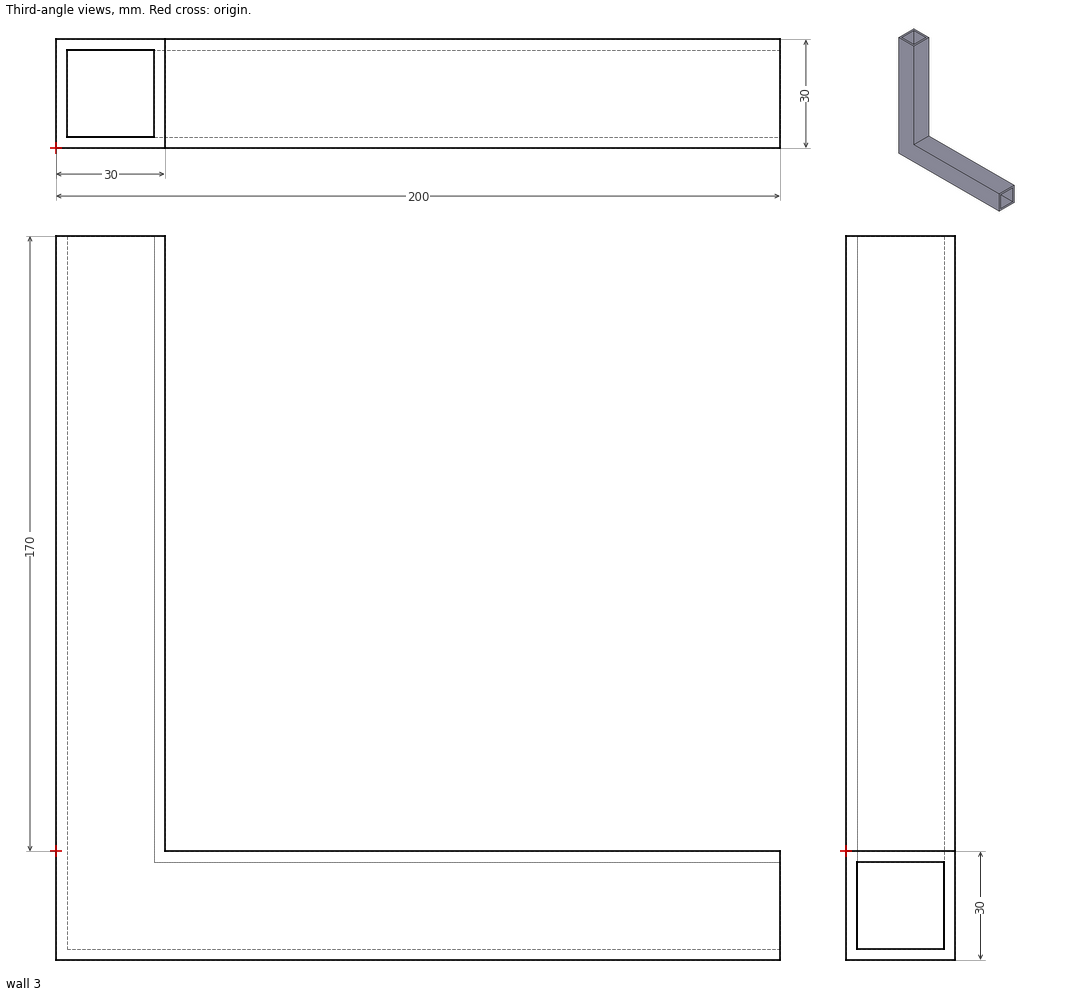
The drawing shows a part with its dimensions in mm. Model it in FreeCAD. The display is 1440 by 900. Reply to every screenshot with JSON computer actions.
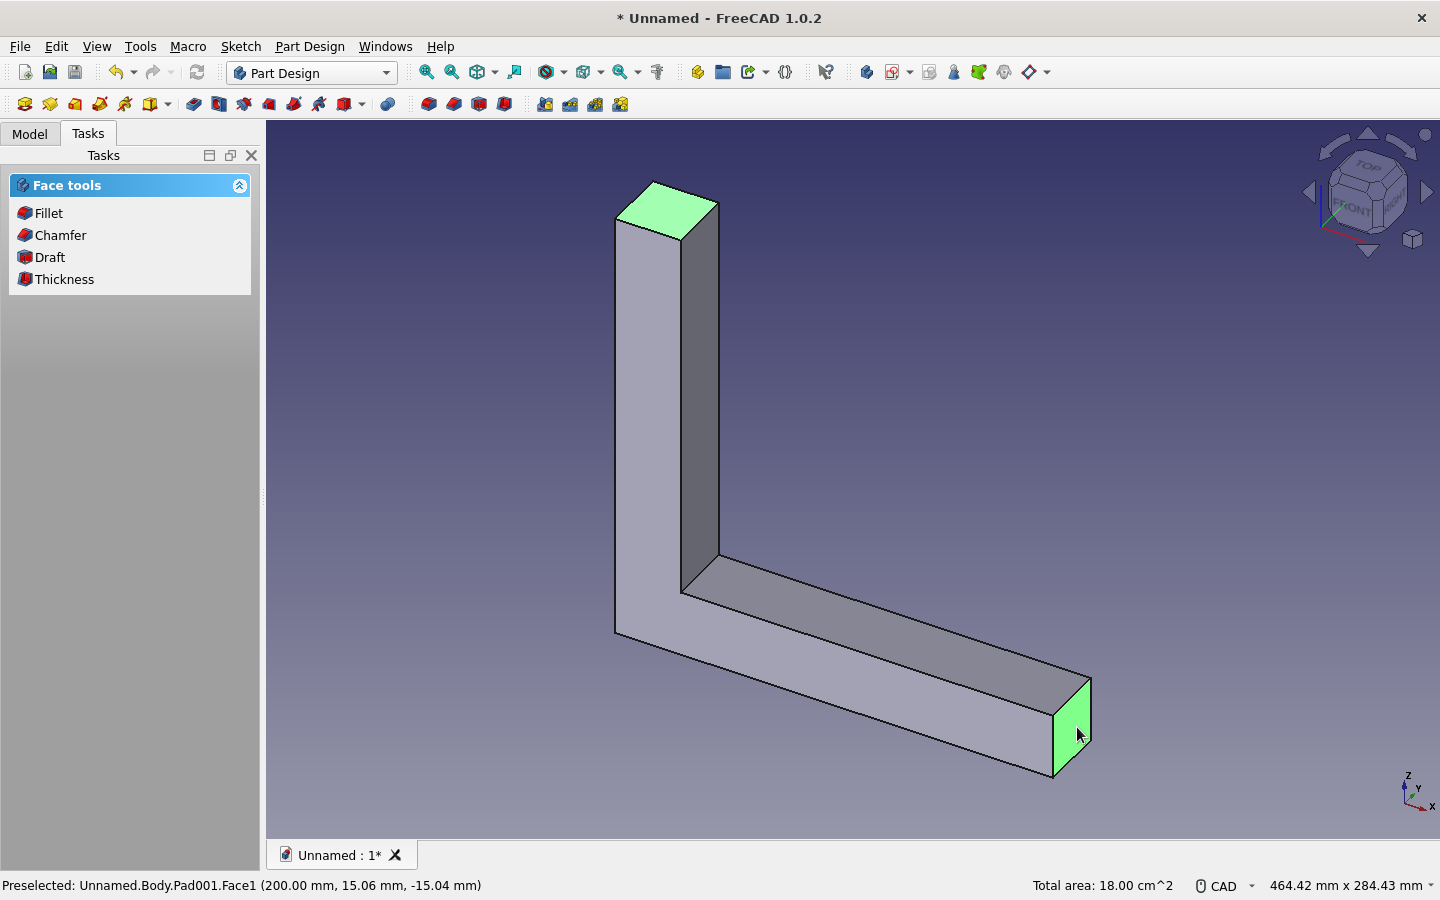
{"action": "left_click", "coordinate": [504, 104]}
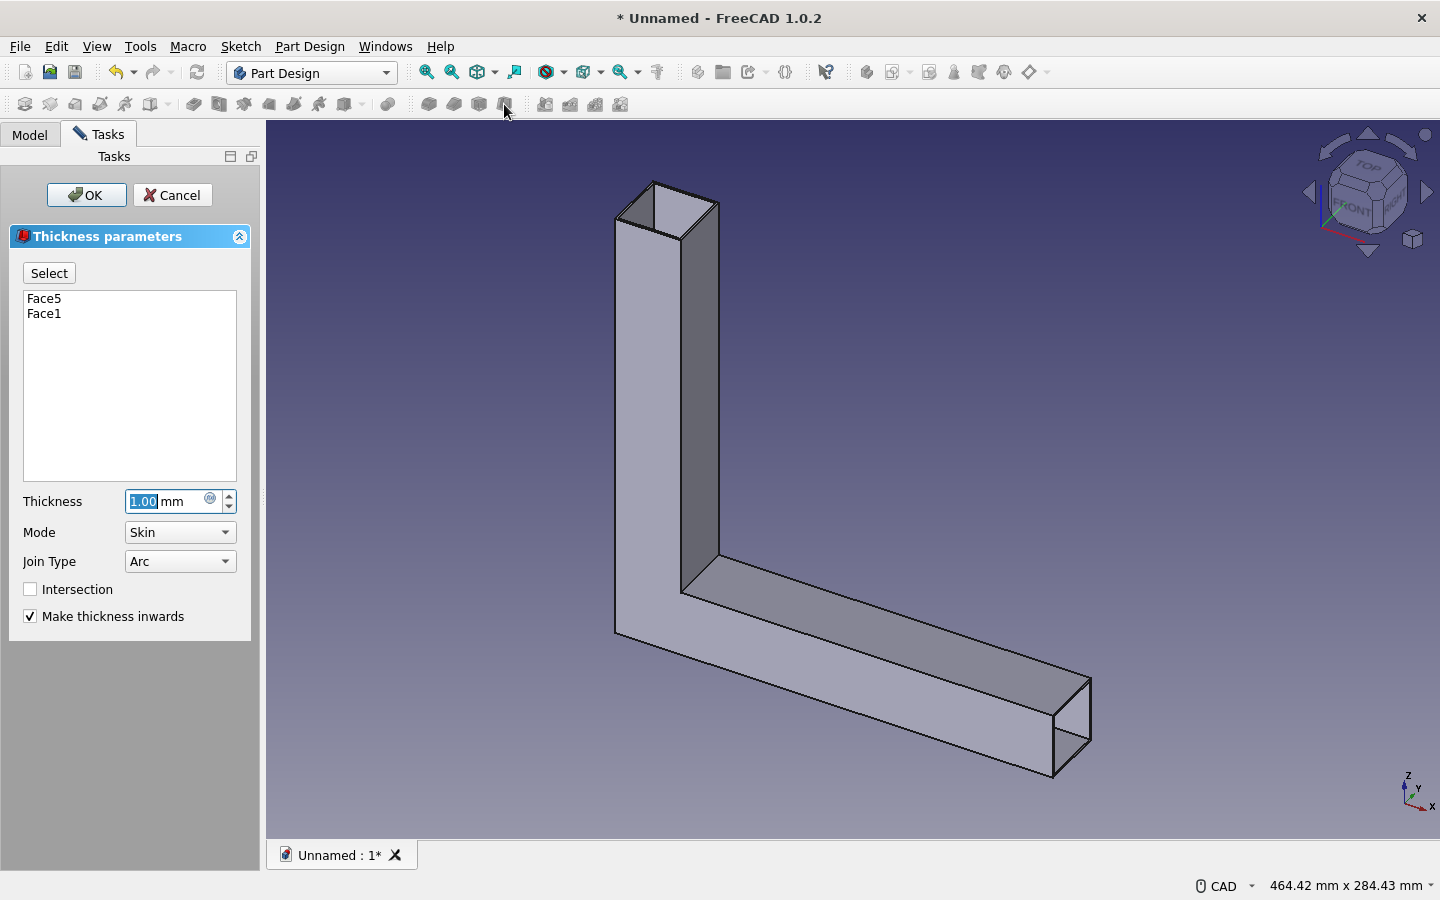
{"action": "type", "text": "3"}
{"action": "key", "text": "Tab"}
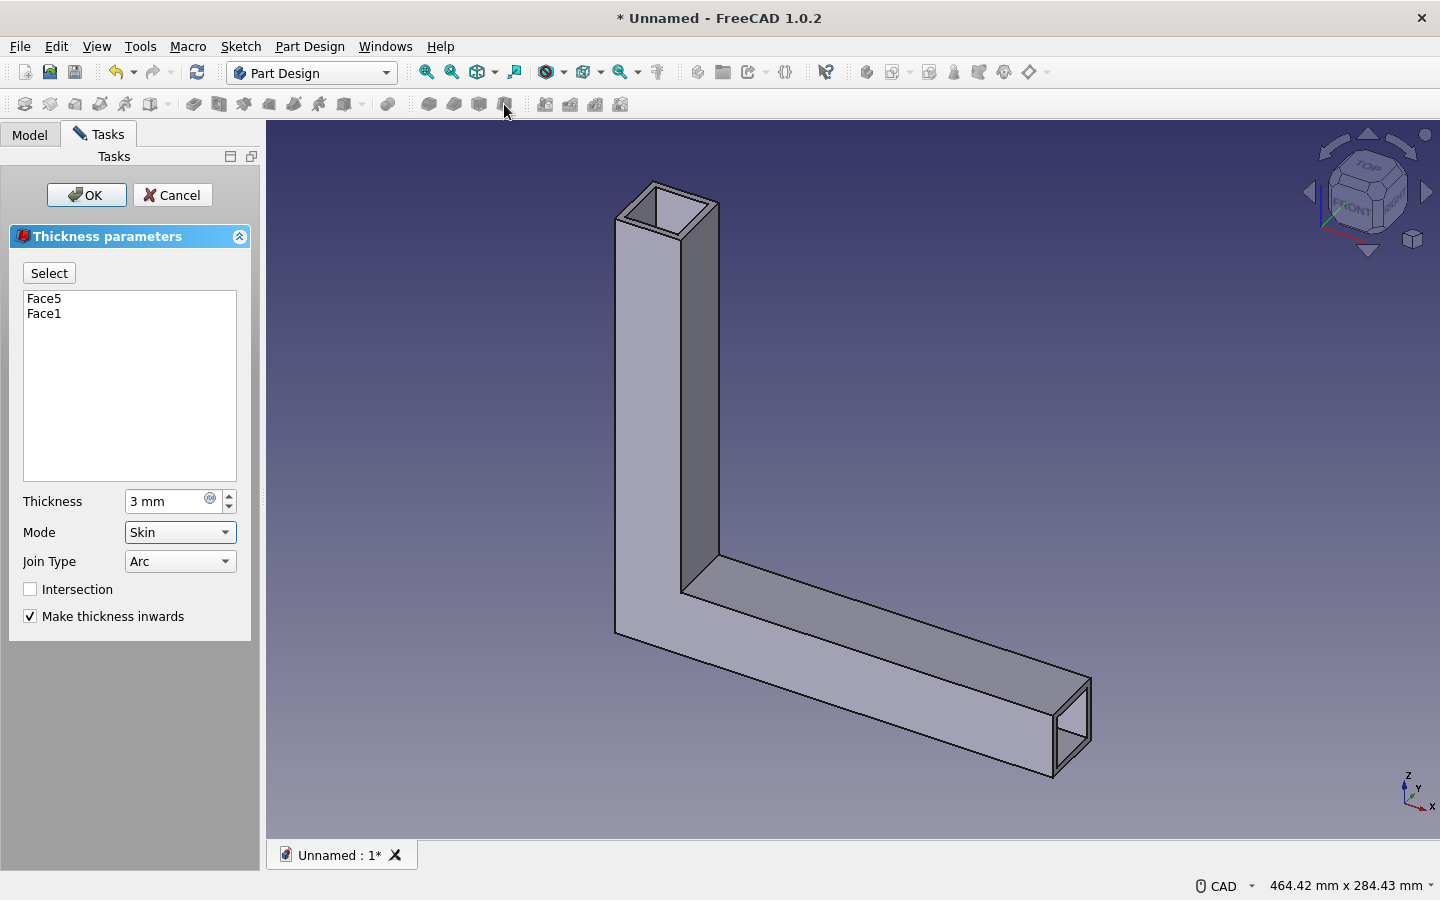
{"action": "left_click", "coordinate": [181, 562]}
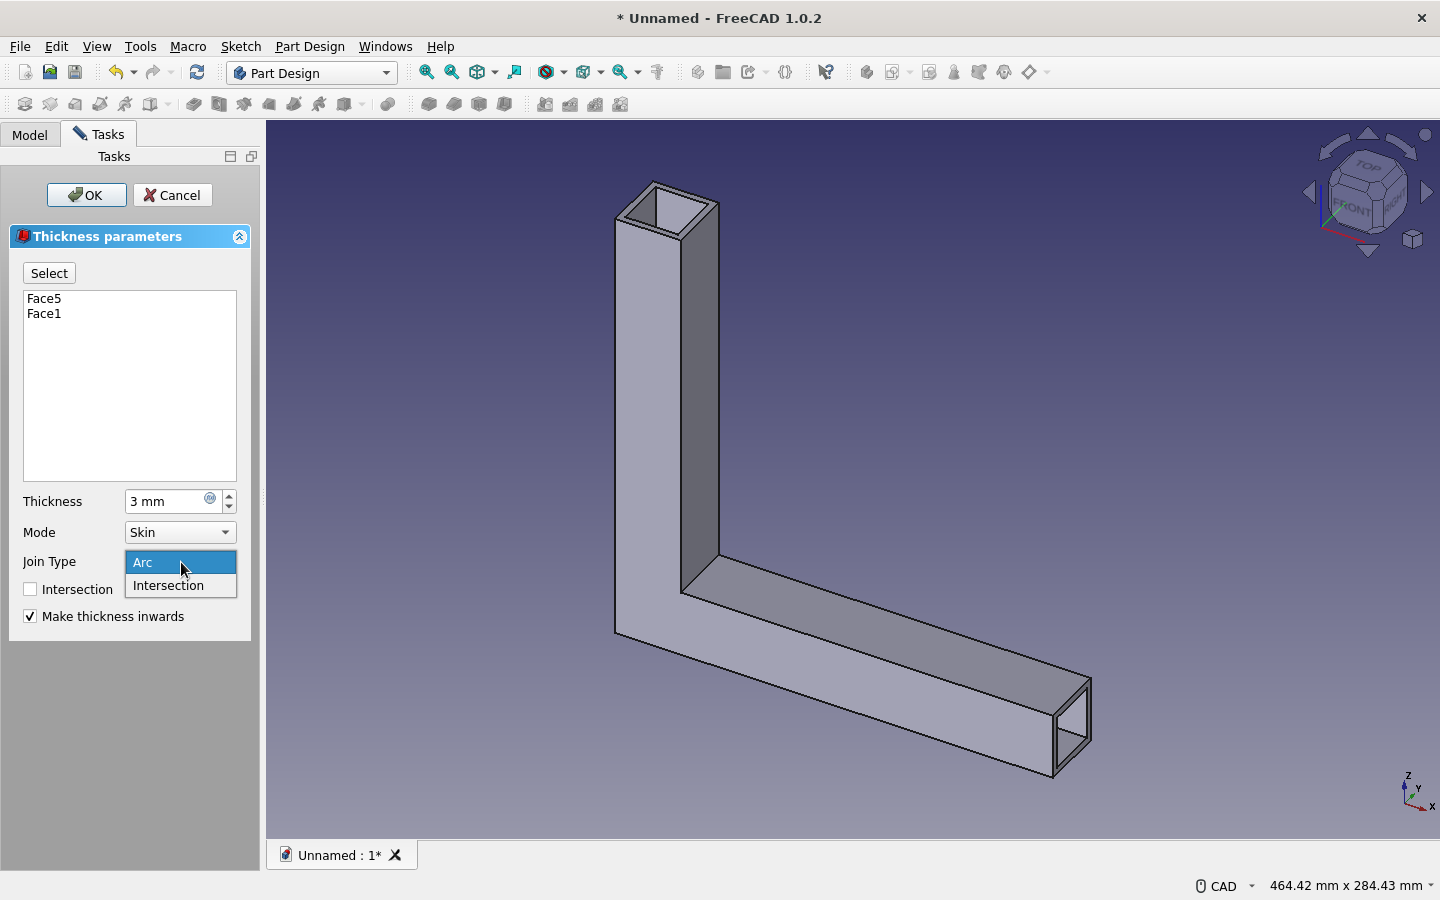
{"action": "left_click", "coordinate": [179, 586]}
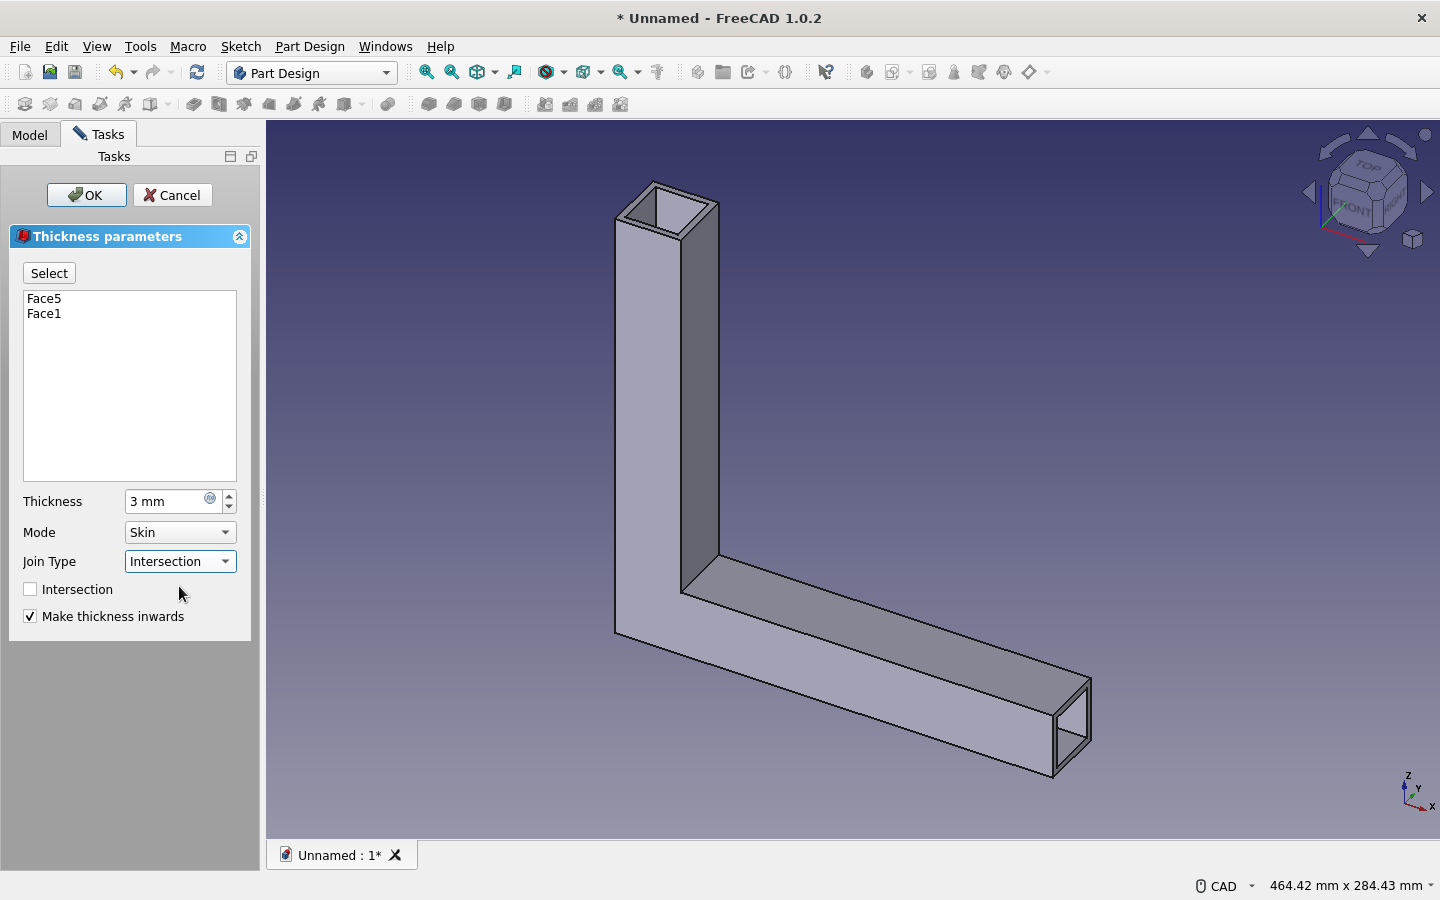
{"action": "left_click", "coordinate": [87, 195]}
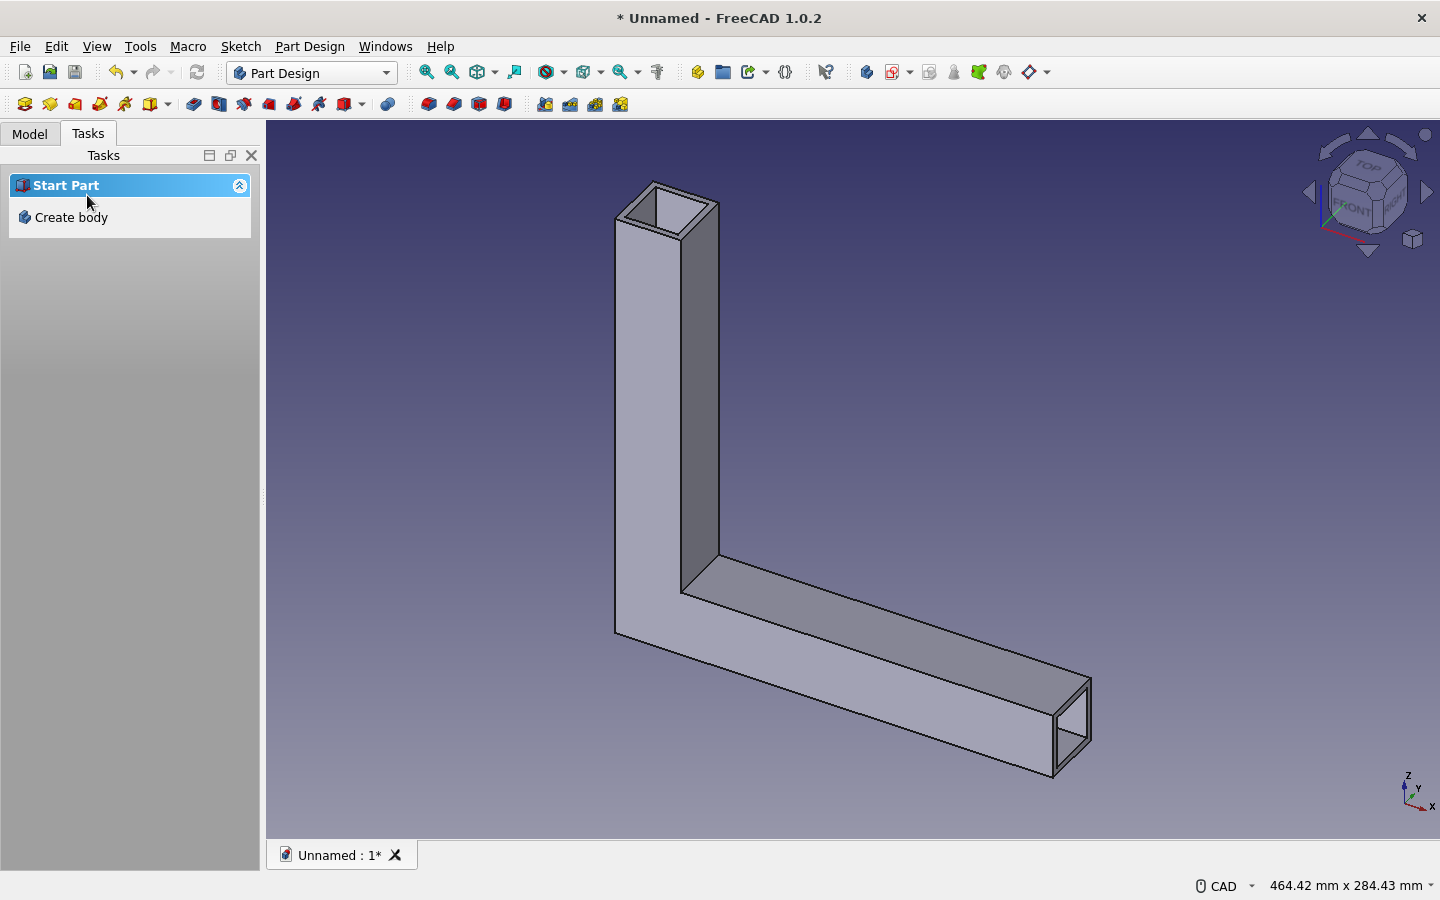
{"action": "key", "text": "0"}